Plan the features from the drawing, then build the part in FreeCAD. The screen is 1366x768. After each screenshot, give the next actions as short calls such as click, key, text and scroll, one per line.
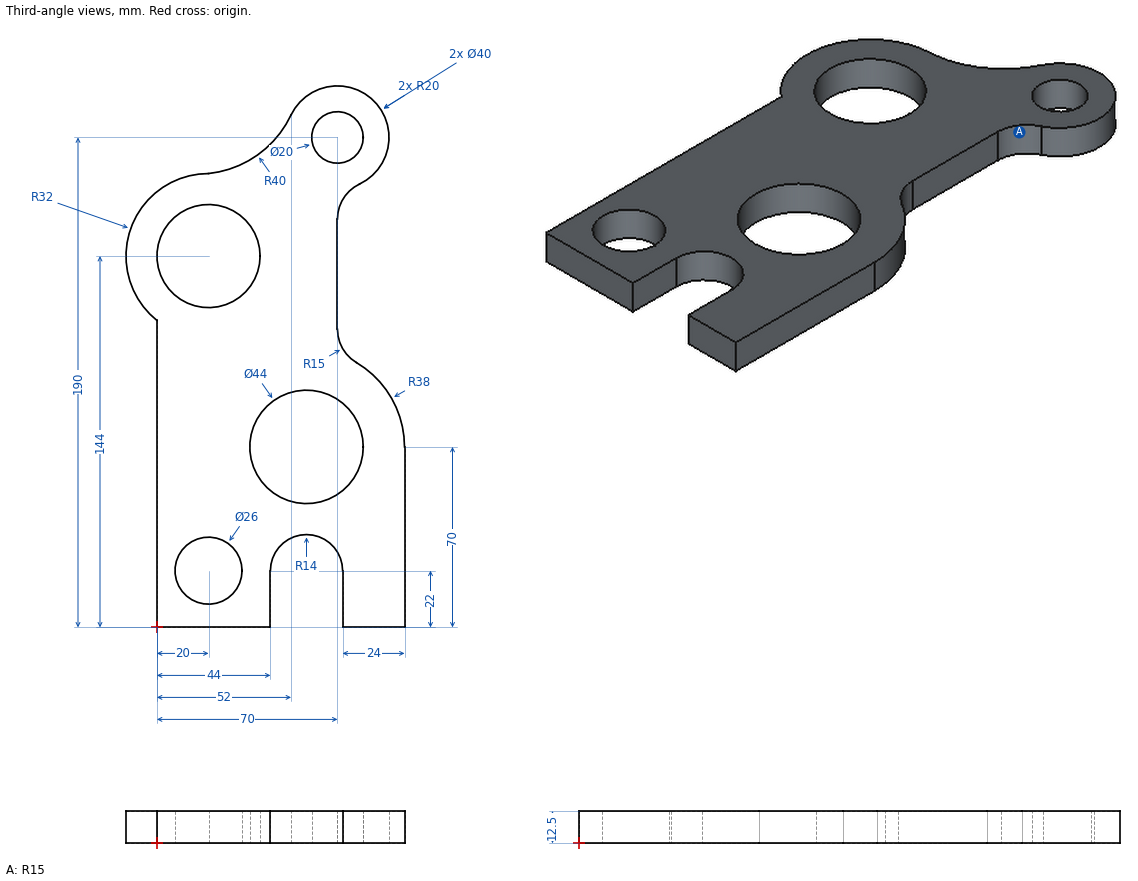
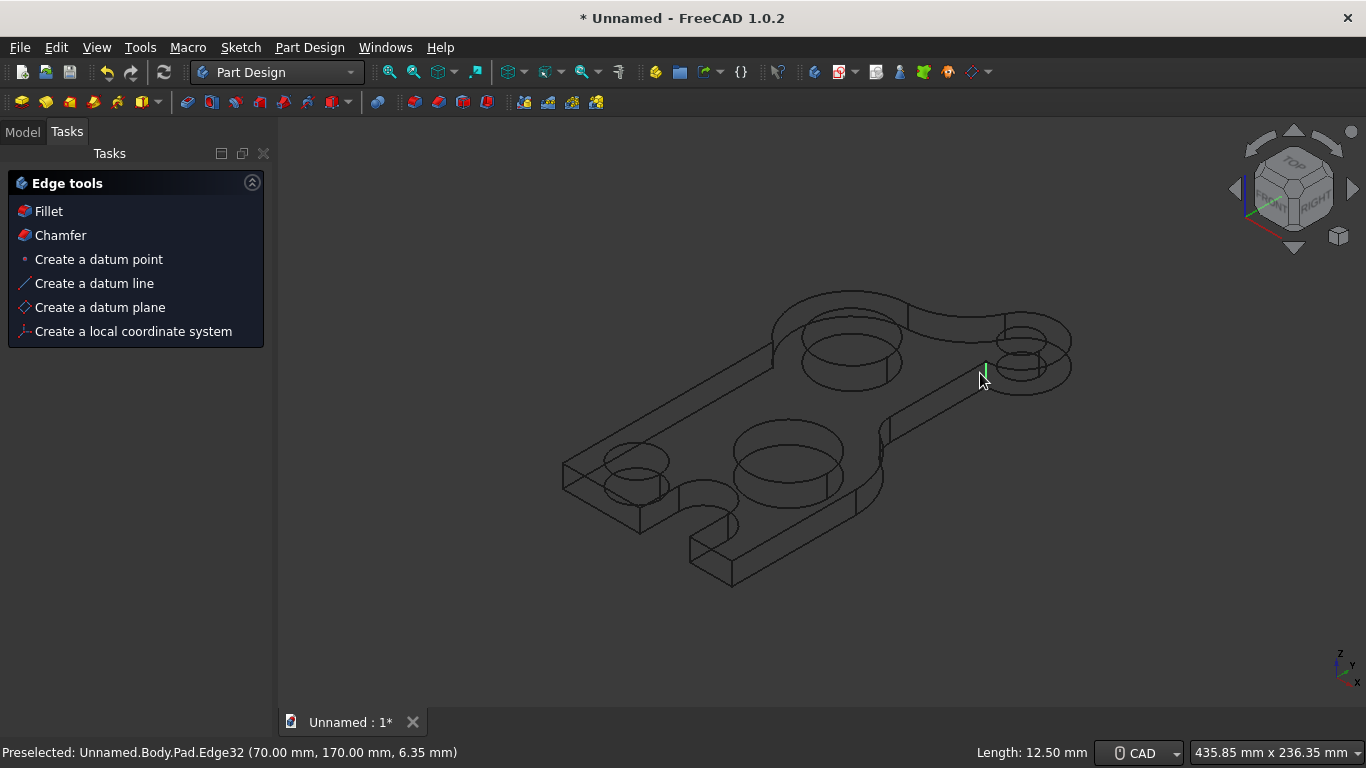
key(v)
key(1)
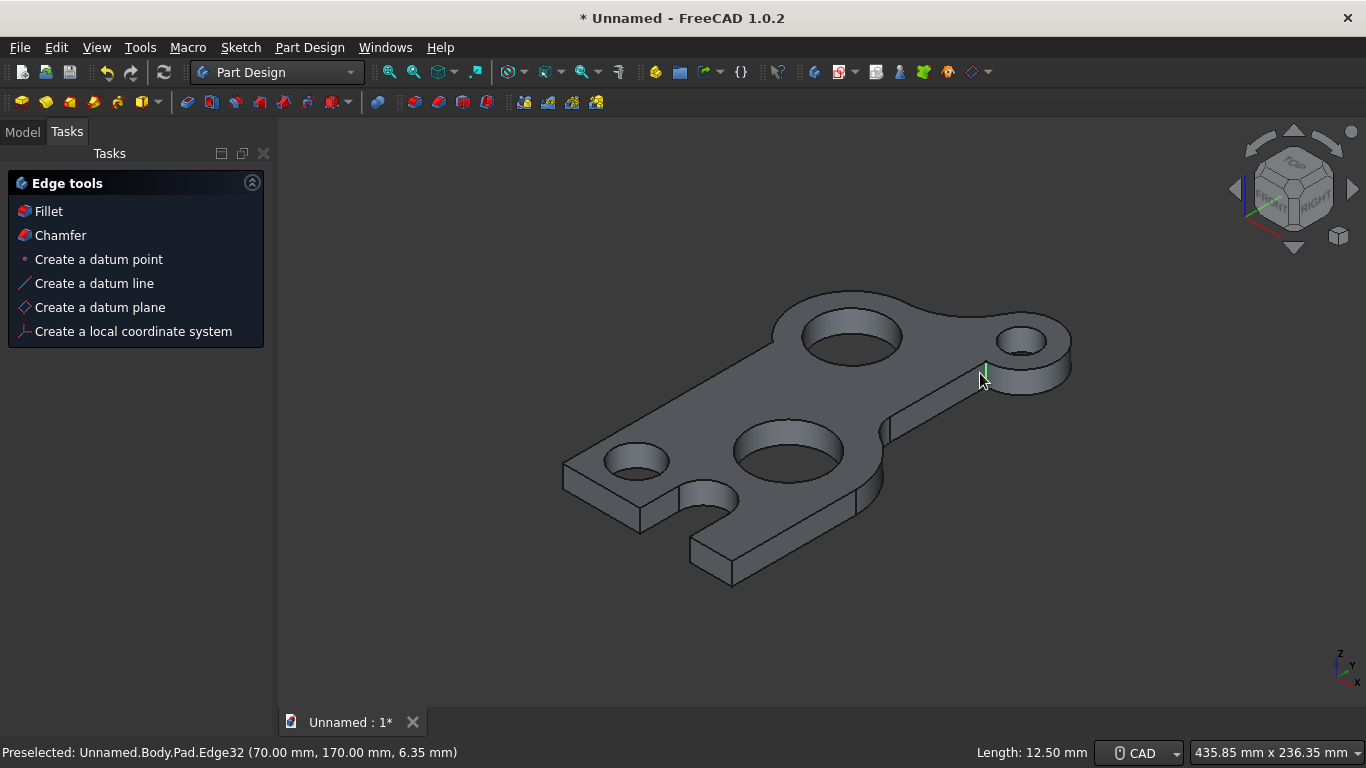
click(416, 102)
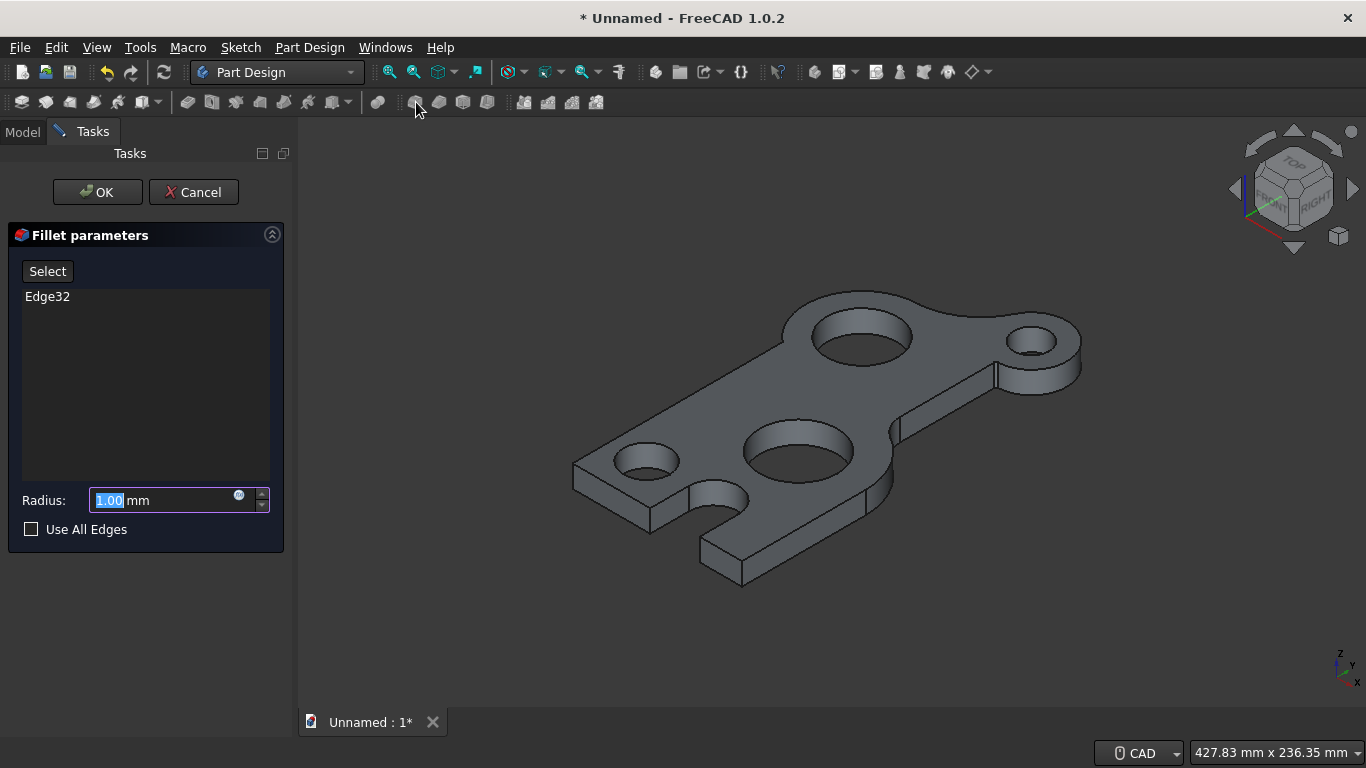
text(15)
key(Tab)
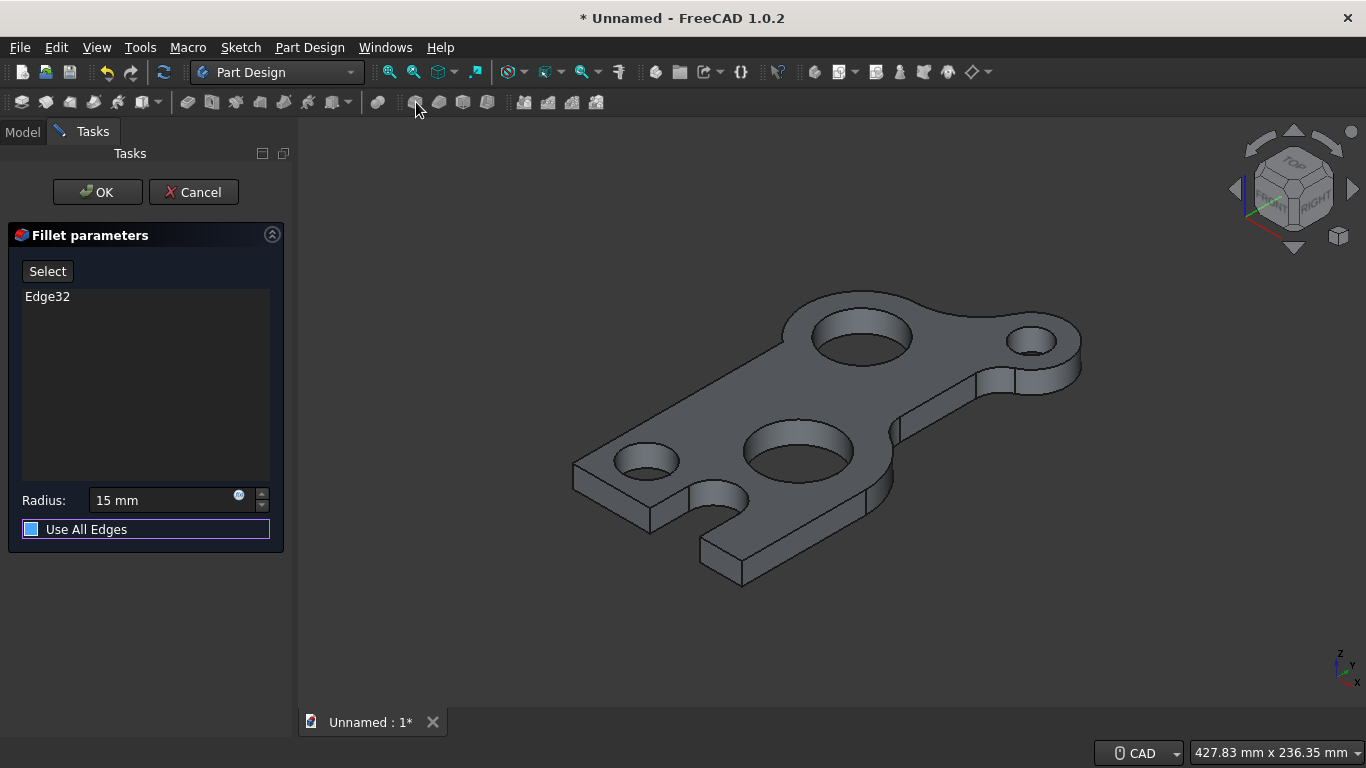
click(98, 192)